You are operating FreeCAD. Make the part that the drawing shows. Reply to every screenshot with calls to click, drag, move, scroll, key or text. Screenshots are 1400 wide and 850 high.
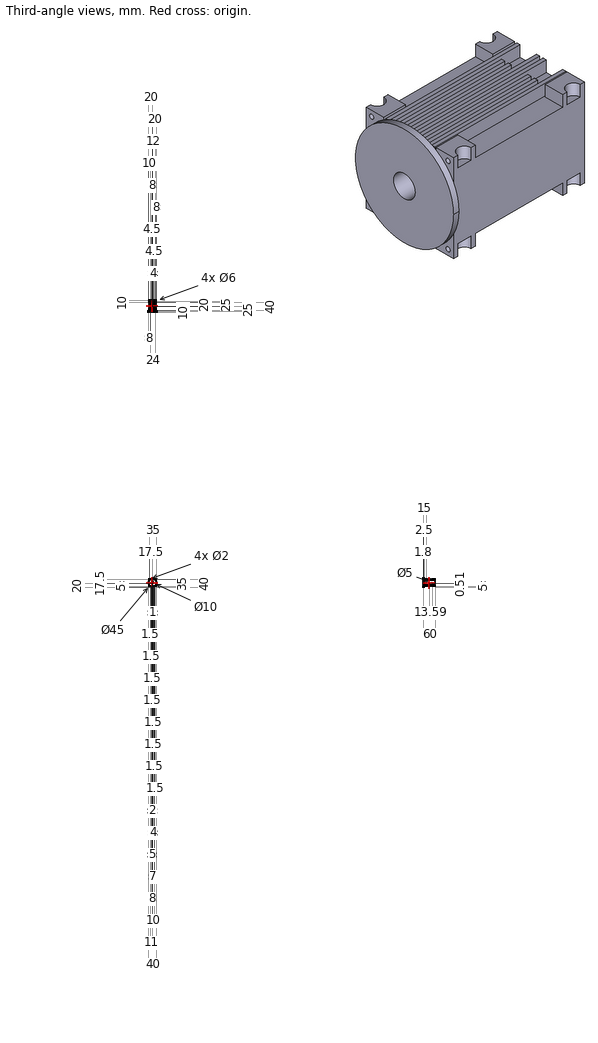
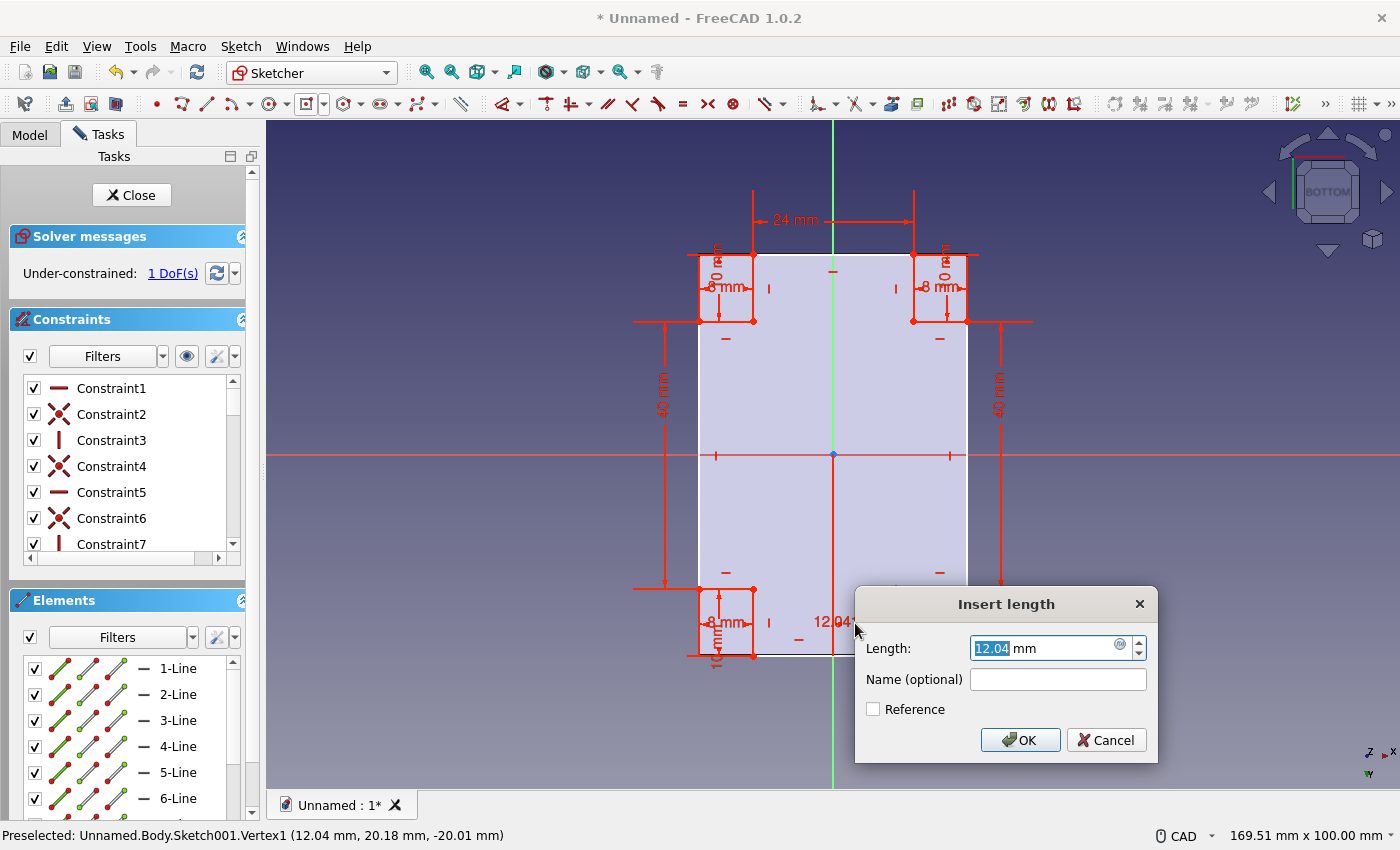
text(12)
key(Return)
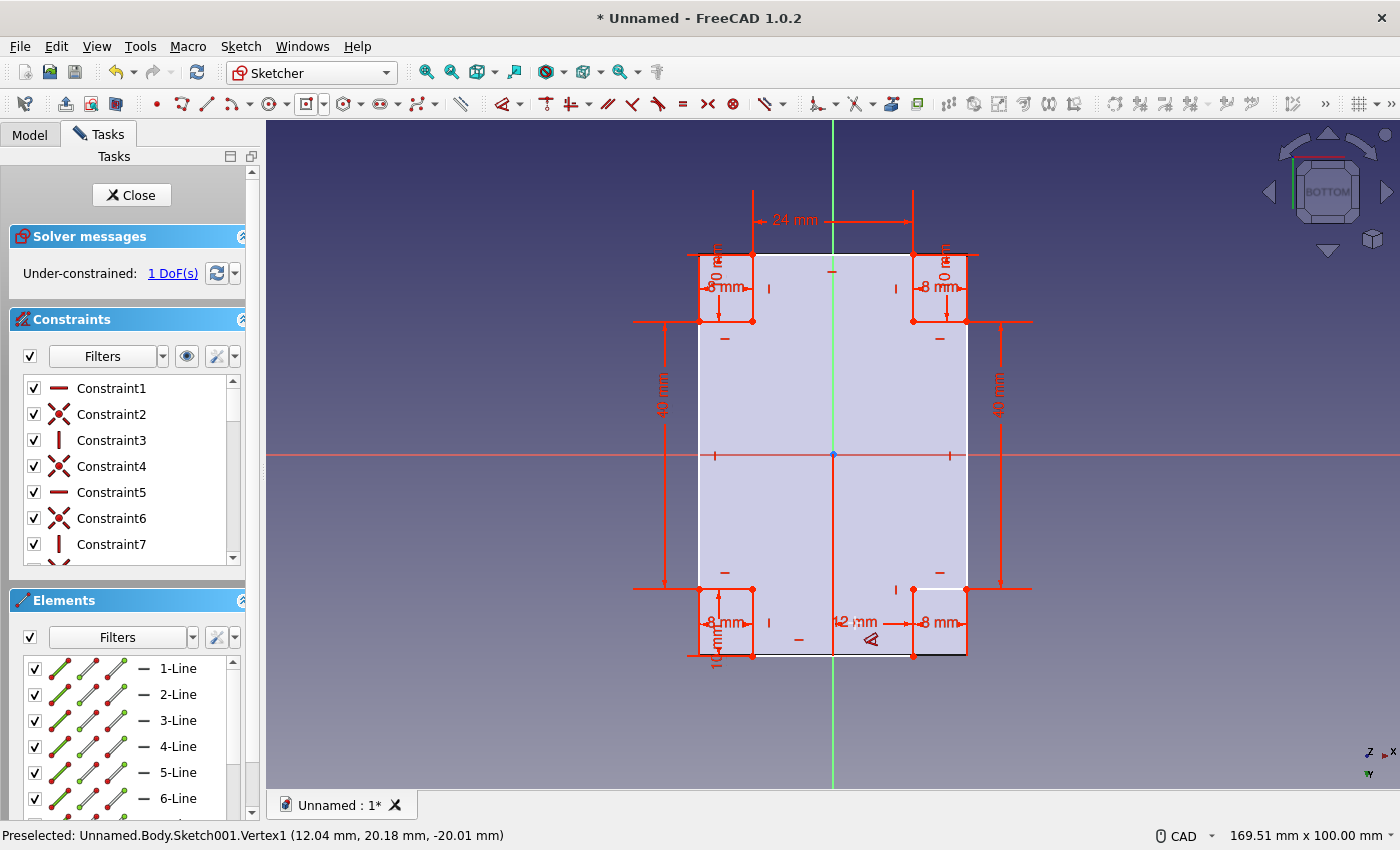
click(913, 589)
click(947, 522)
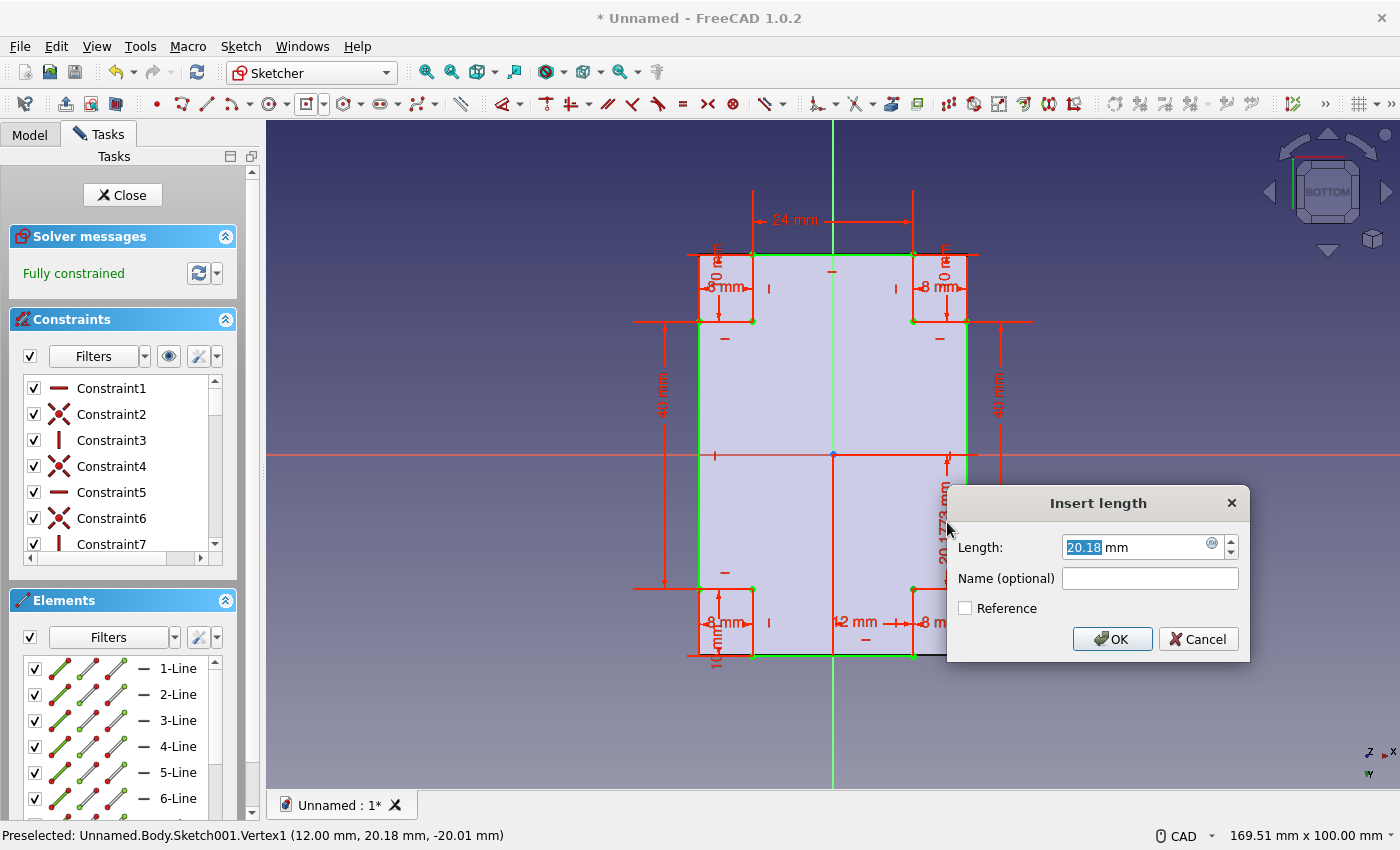
text(20)
key(Return)
key(Escape)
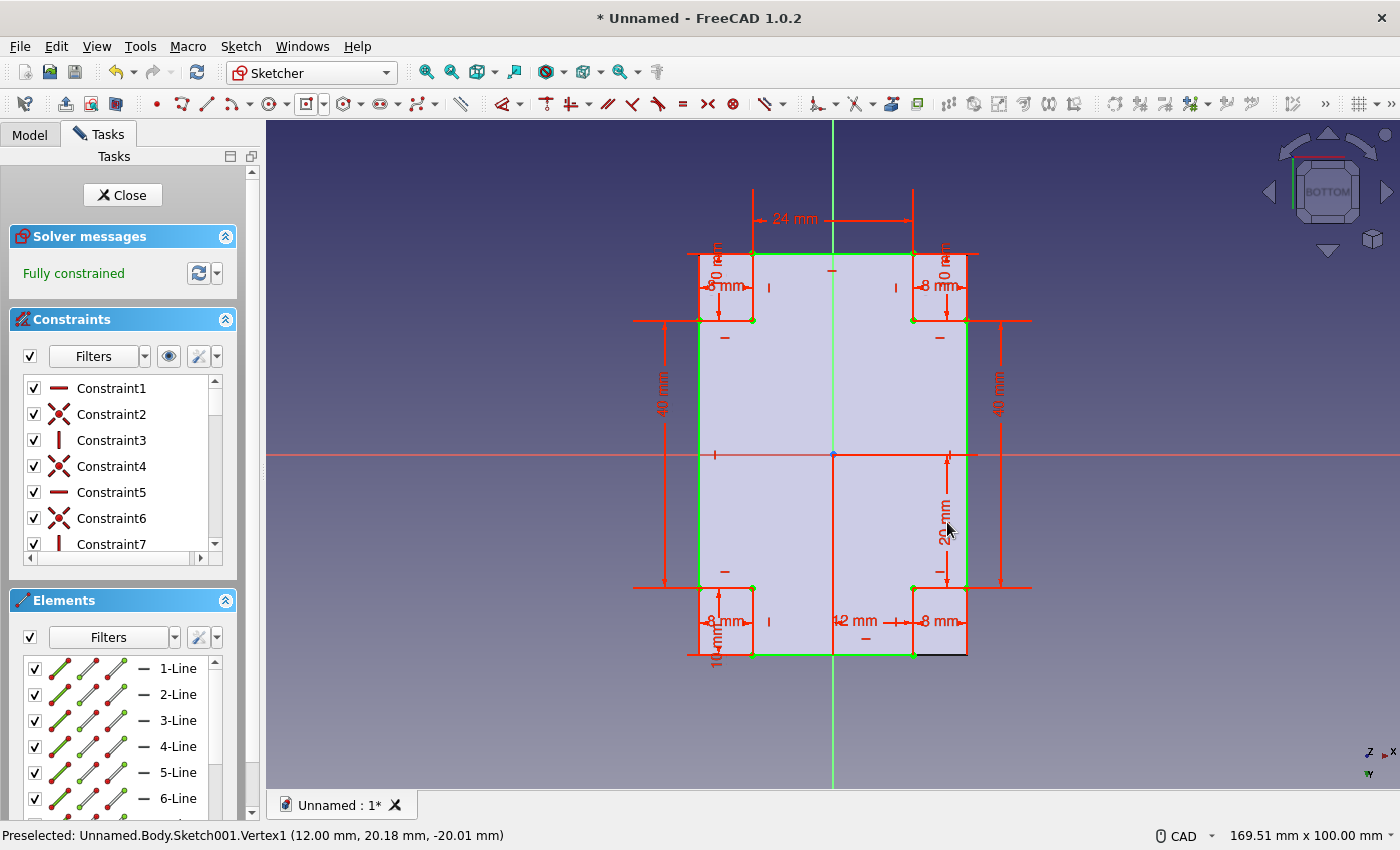
click(123, 195)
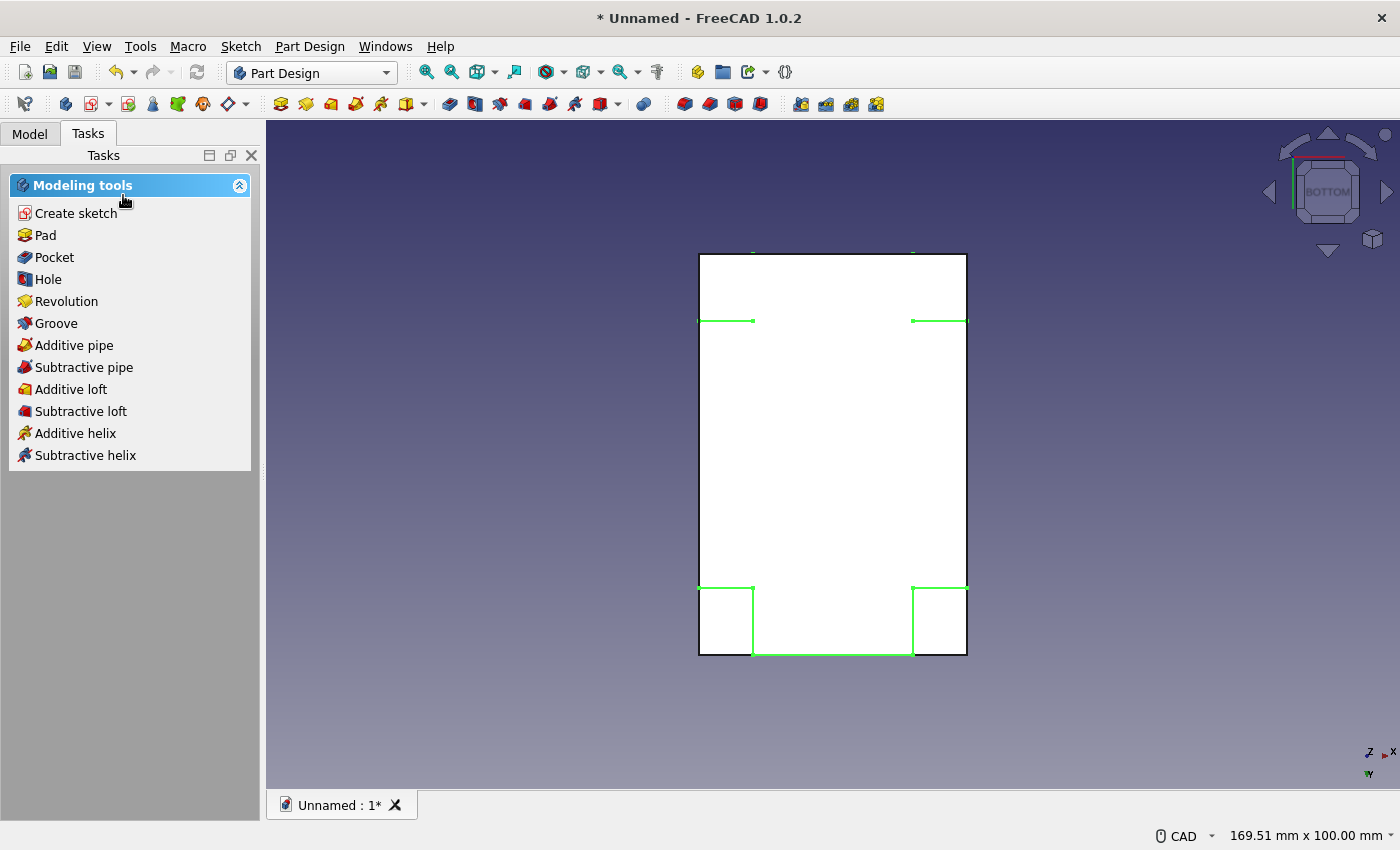
click(450, 104)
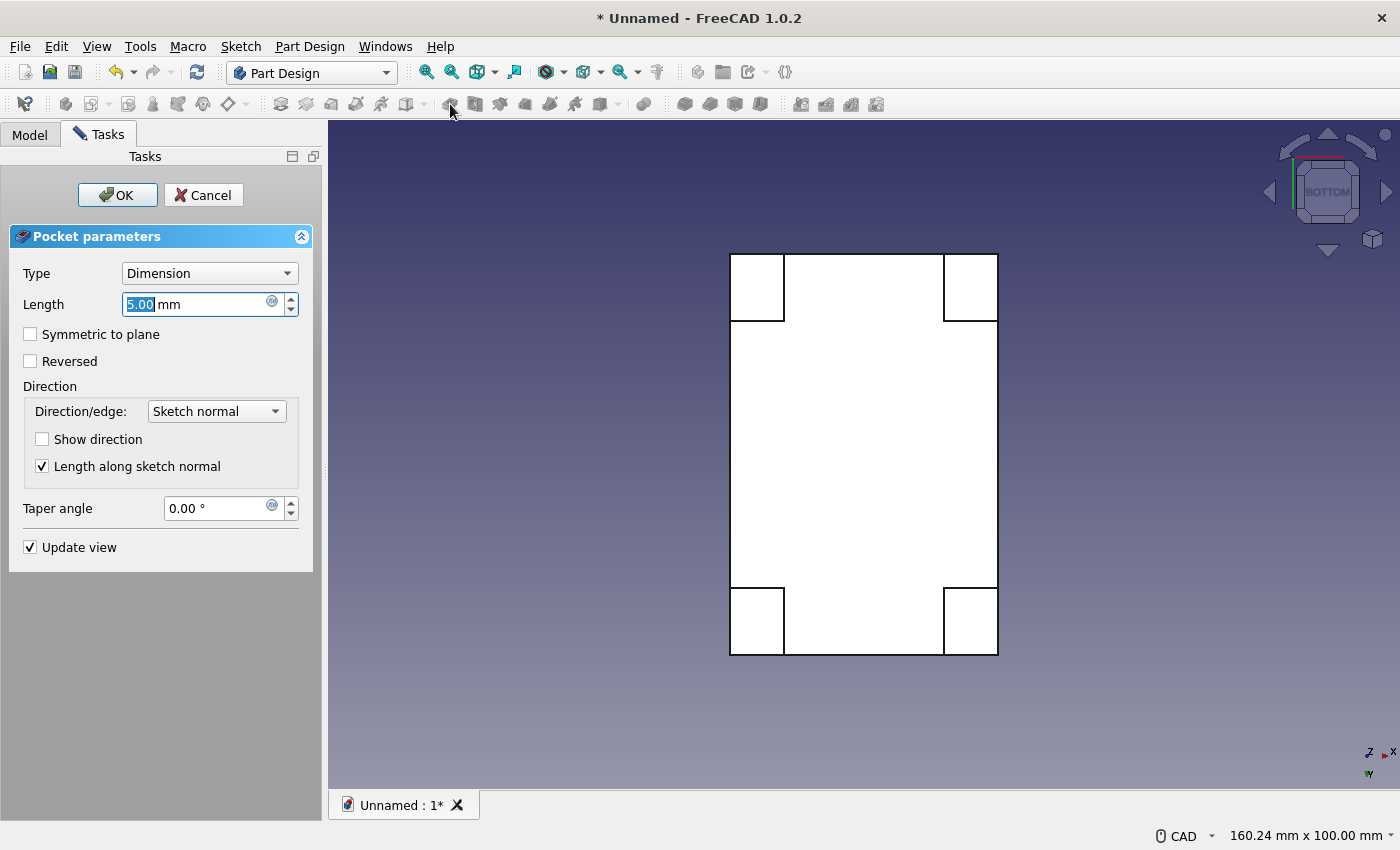
text(5)
key(Tab)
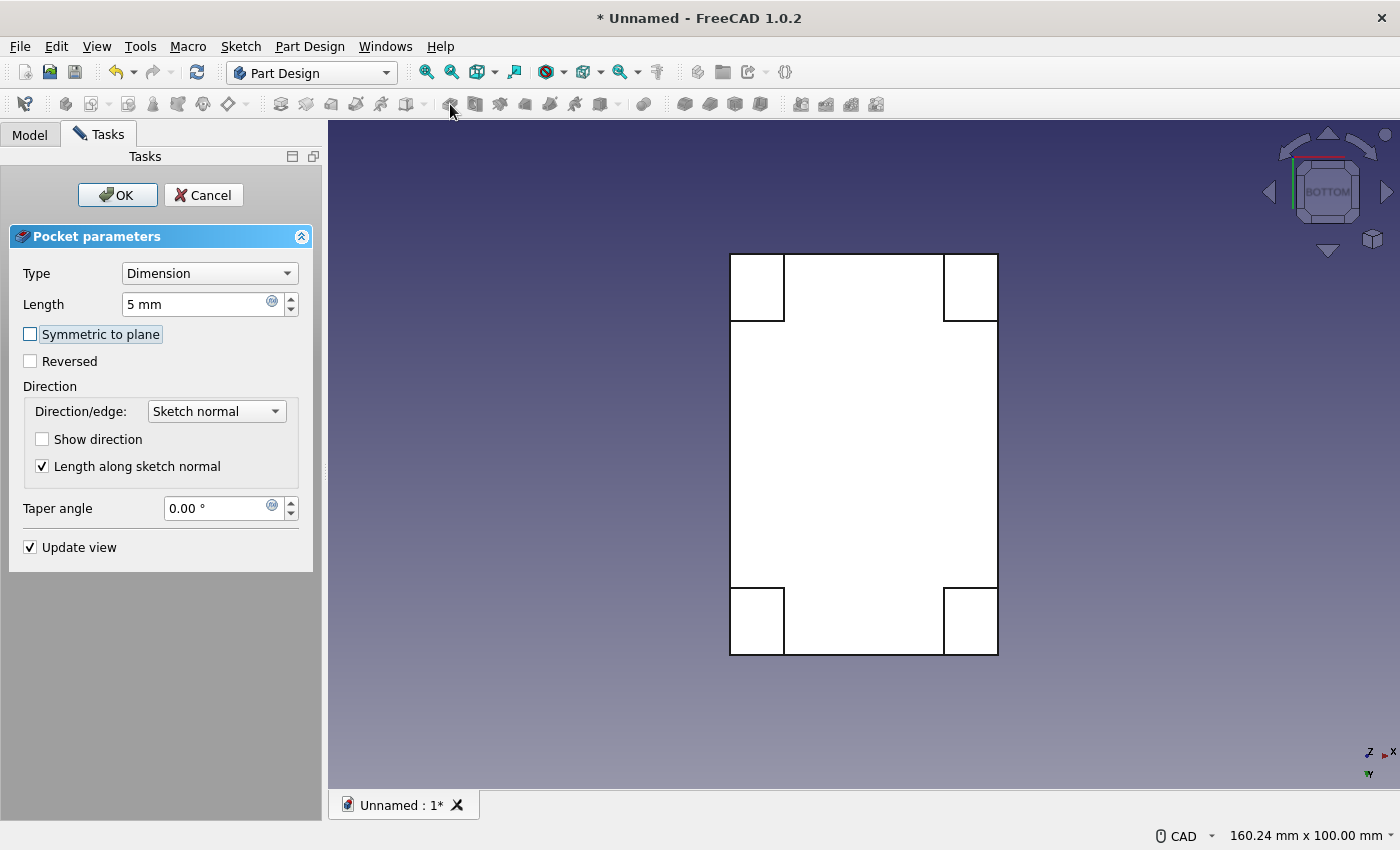
click(118, 195)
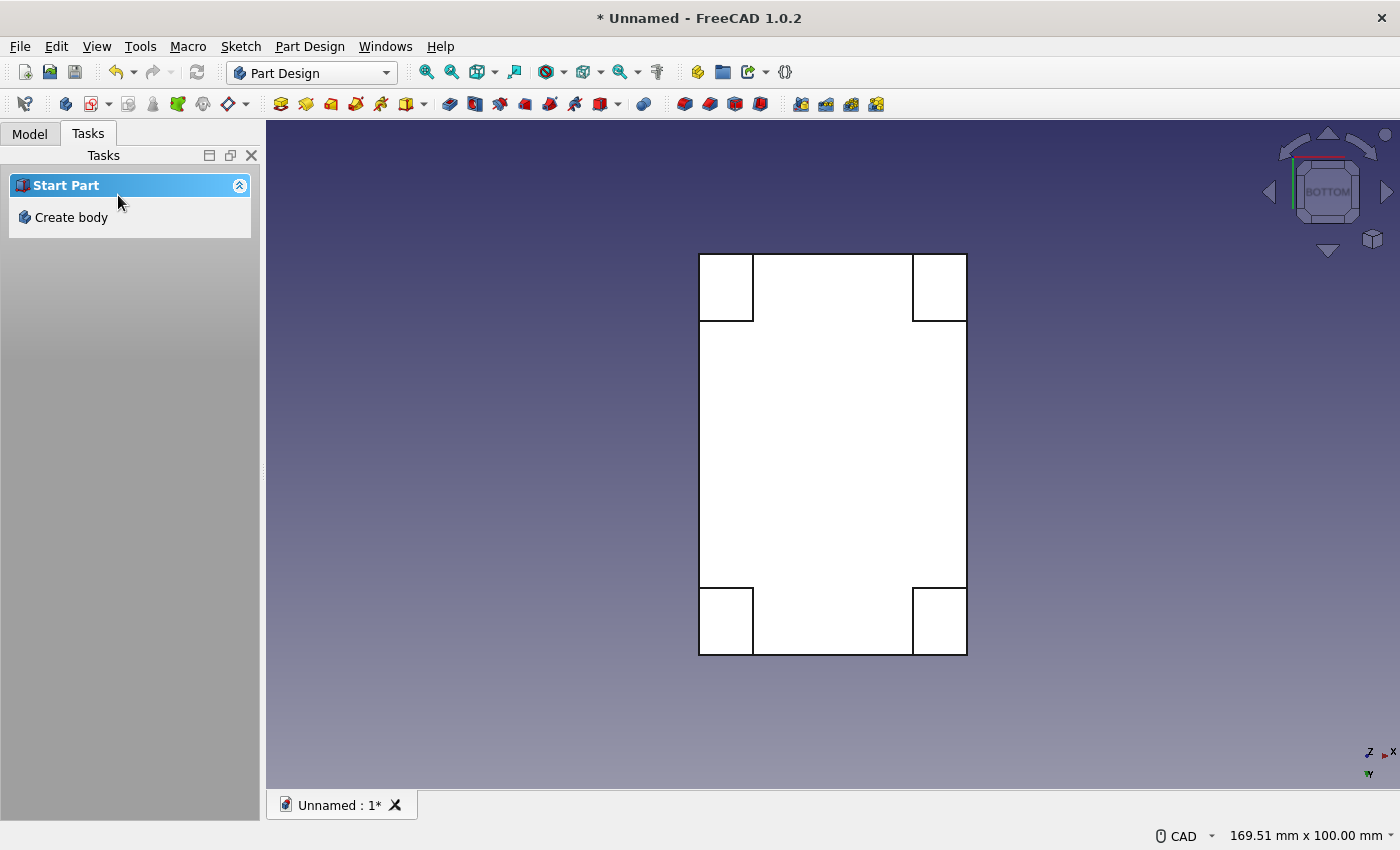
click(30, 134)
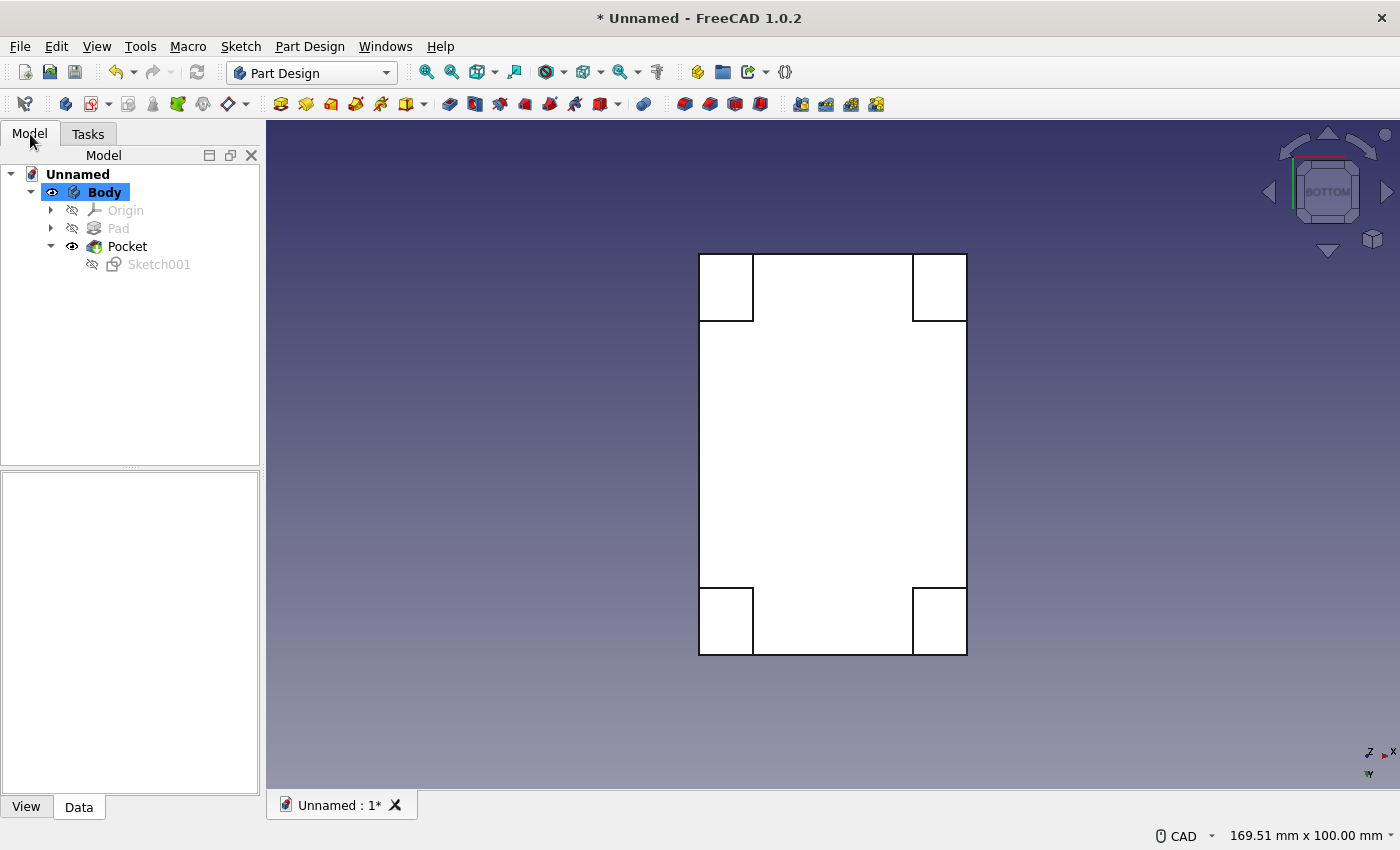
click(117, 246)